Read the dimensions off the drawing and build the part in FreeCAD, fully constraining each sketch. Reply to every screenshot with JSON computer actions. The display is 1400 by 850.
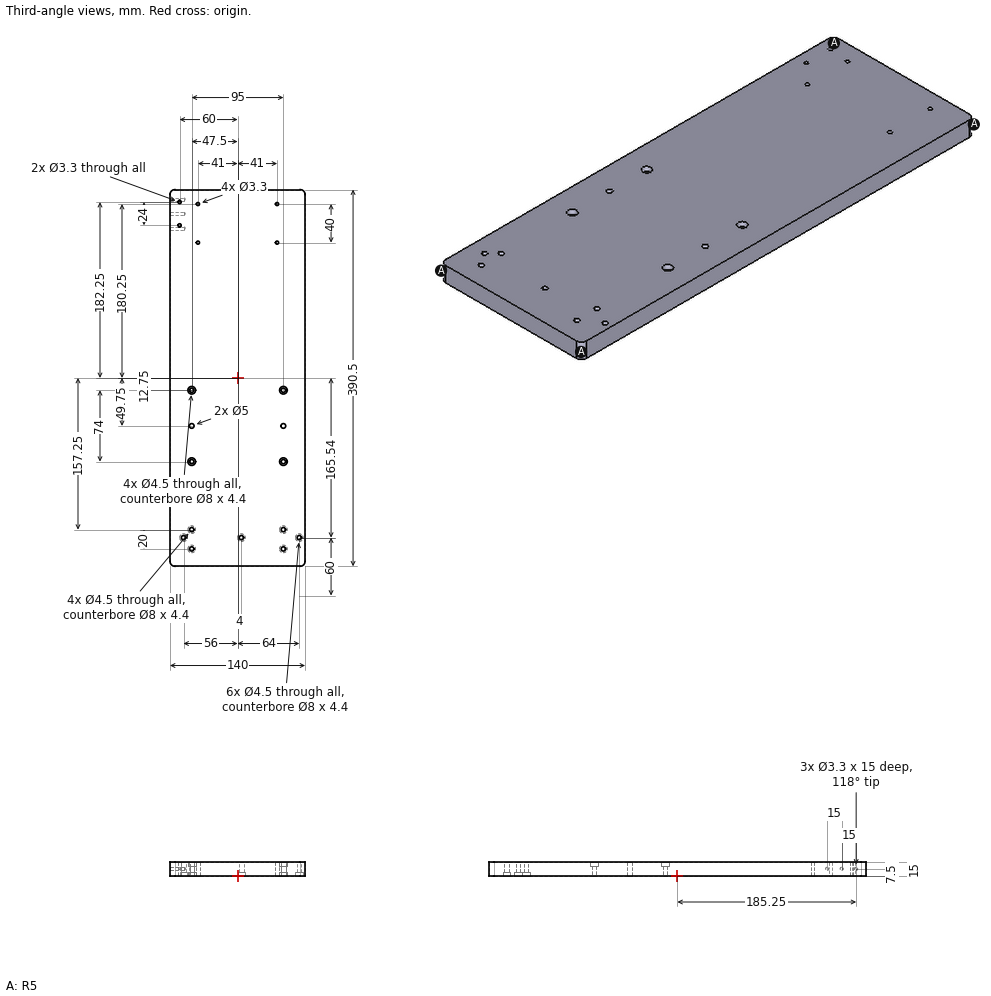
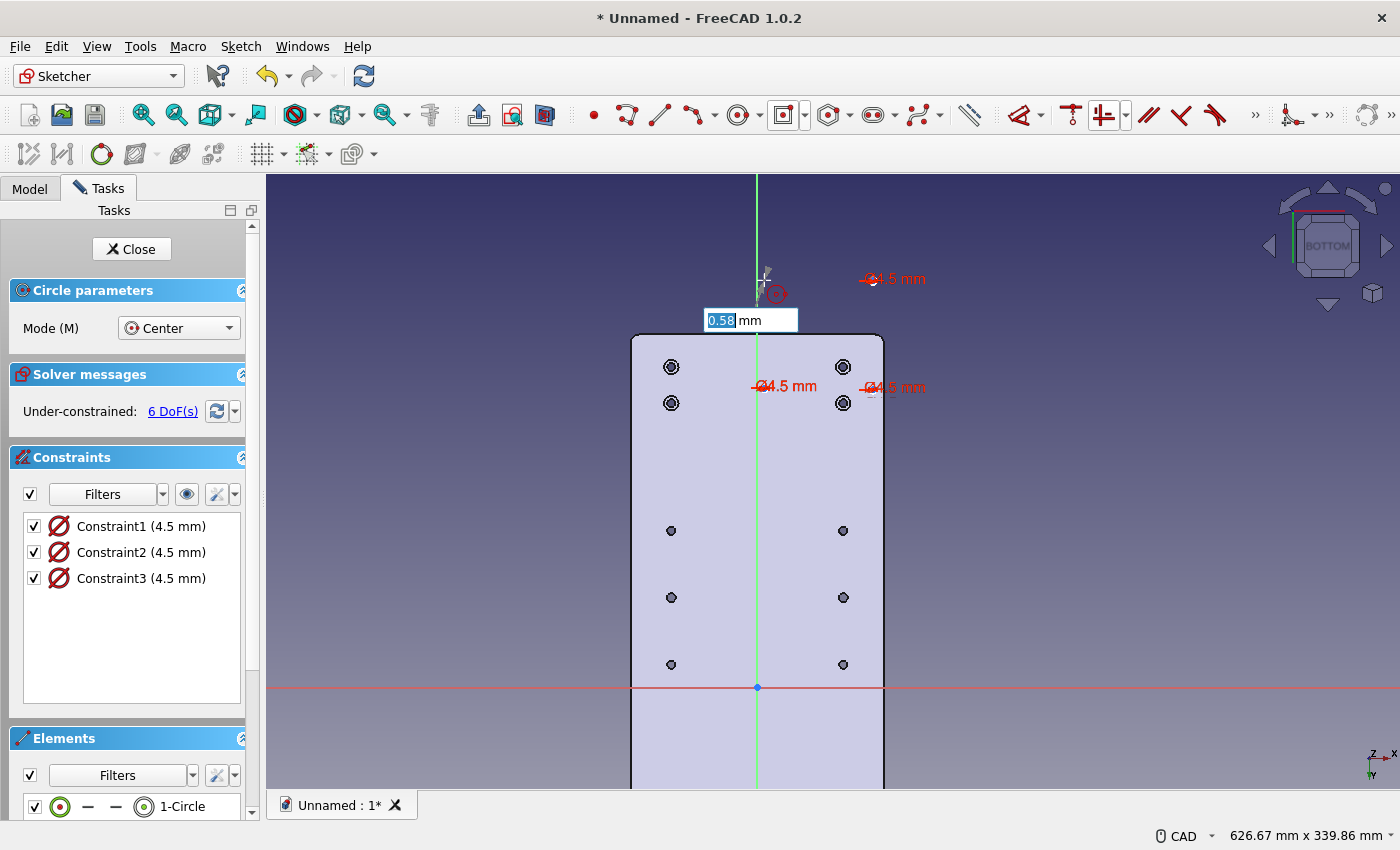
{"action": "scroll", "coordinate": [767, 277], "scroll_direction": "up", "scroll_amount": 3}
{"action": "mouse_move", "coordinate": [767, 276]}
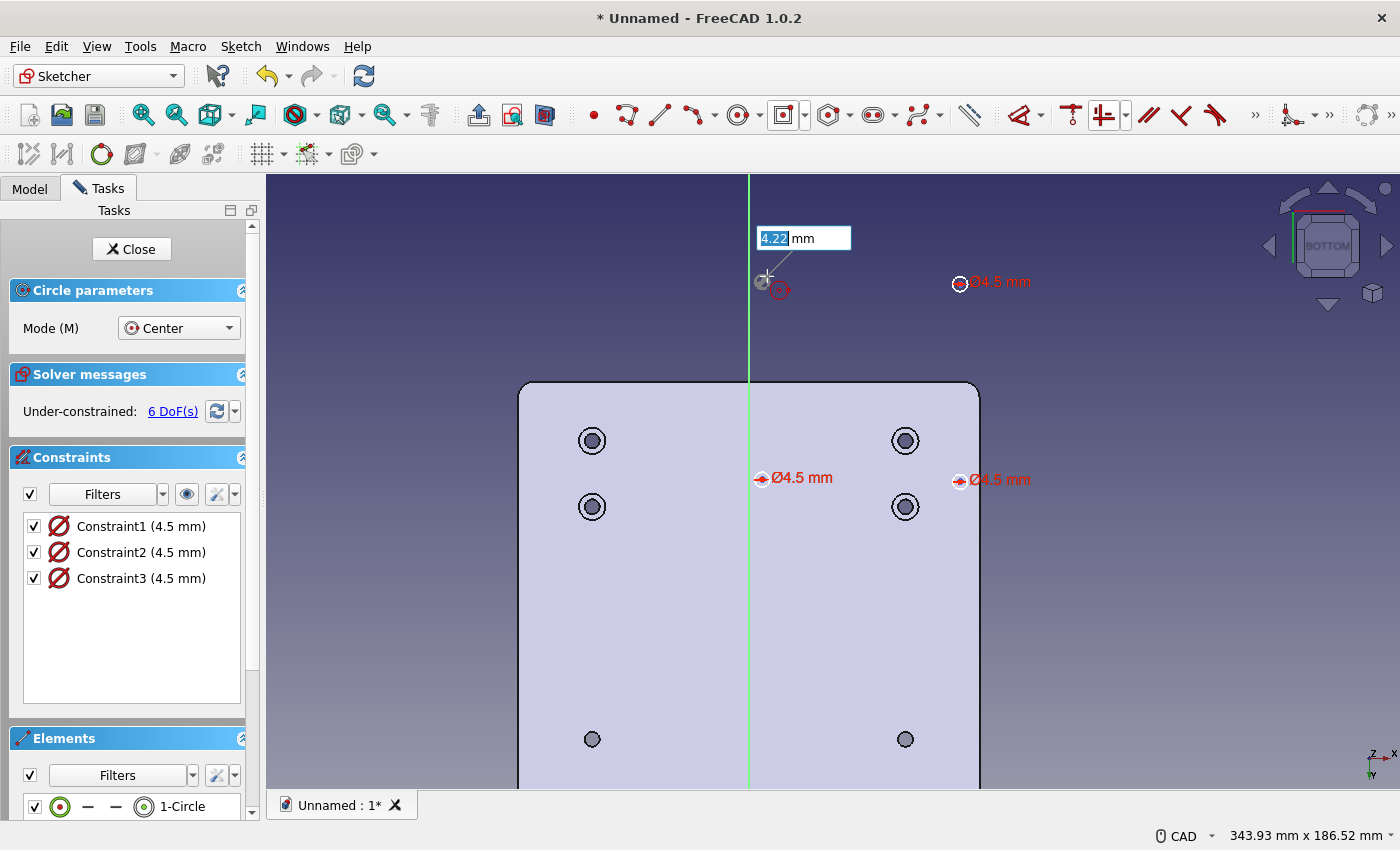
{"action": "type", "text": "4.5"}
{"action": "key", "text": "Return"}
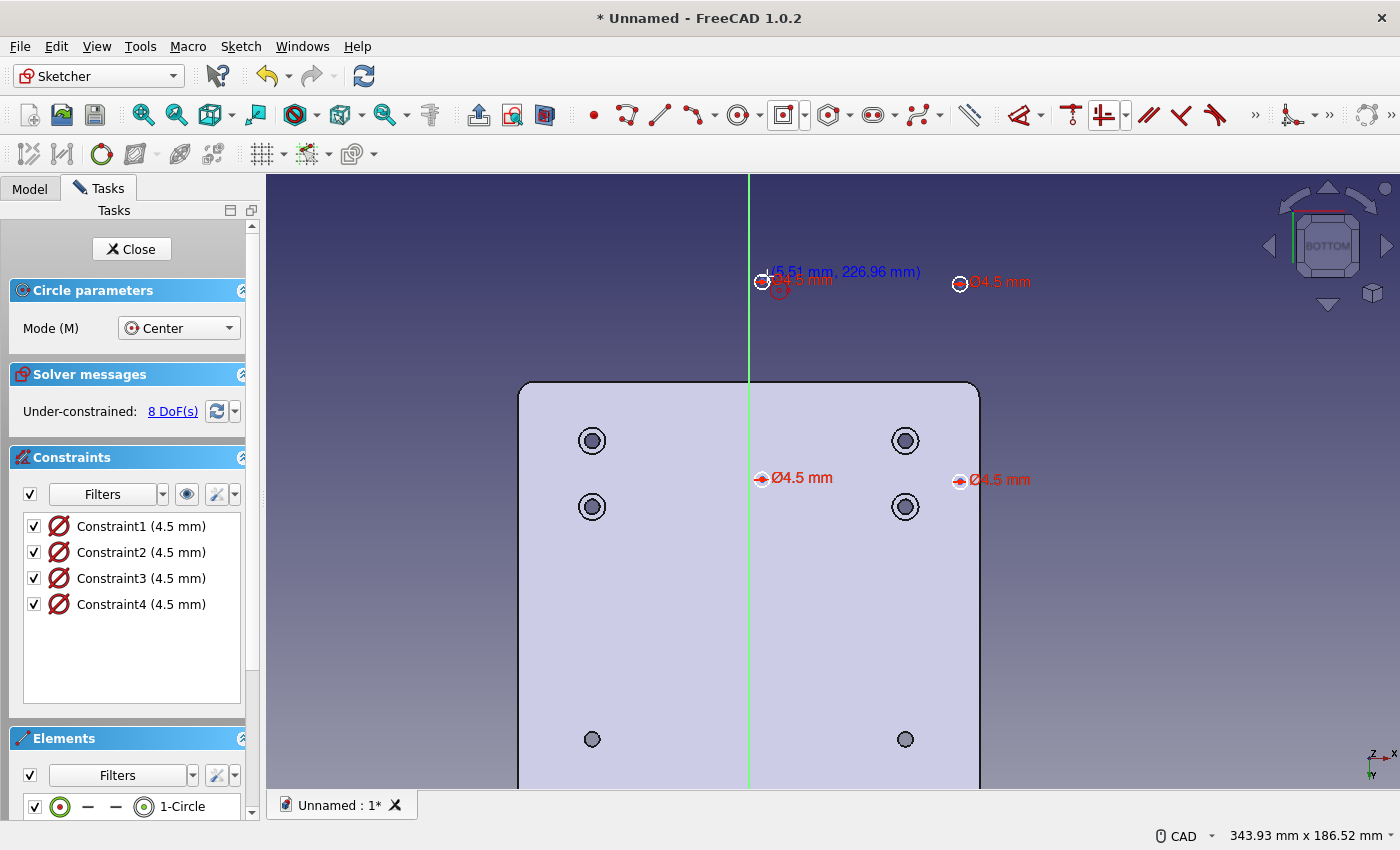
{"action": "scroll", "coordinate": [564, 480], "scroll_direction": "up", "scroll_amount": 6}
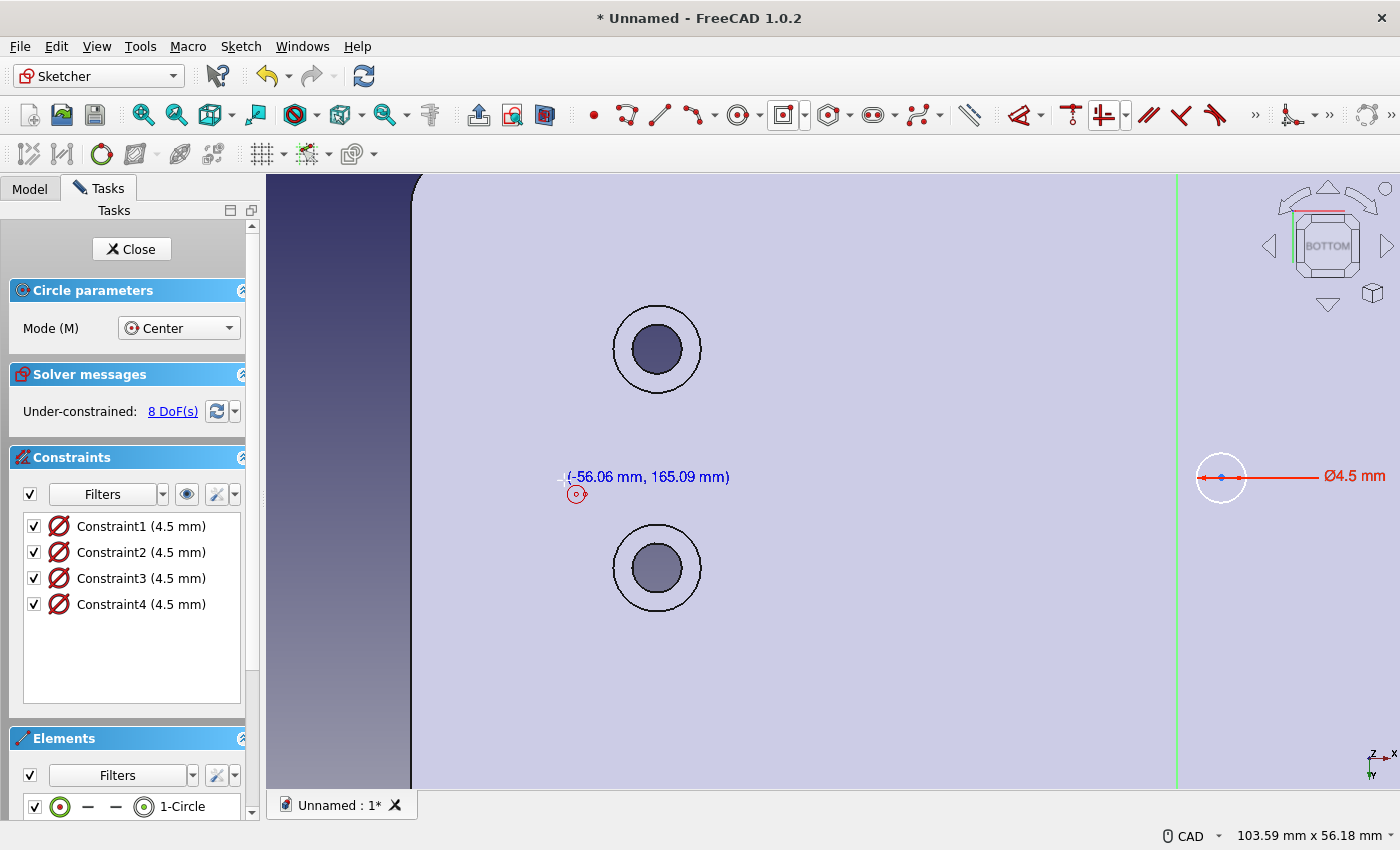
{"action": "scroll", "coordinate": [674, 370], "scroll_direction": "down", "scroll_amount": 9}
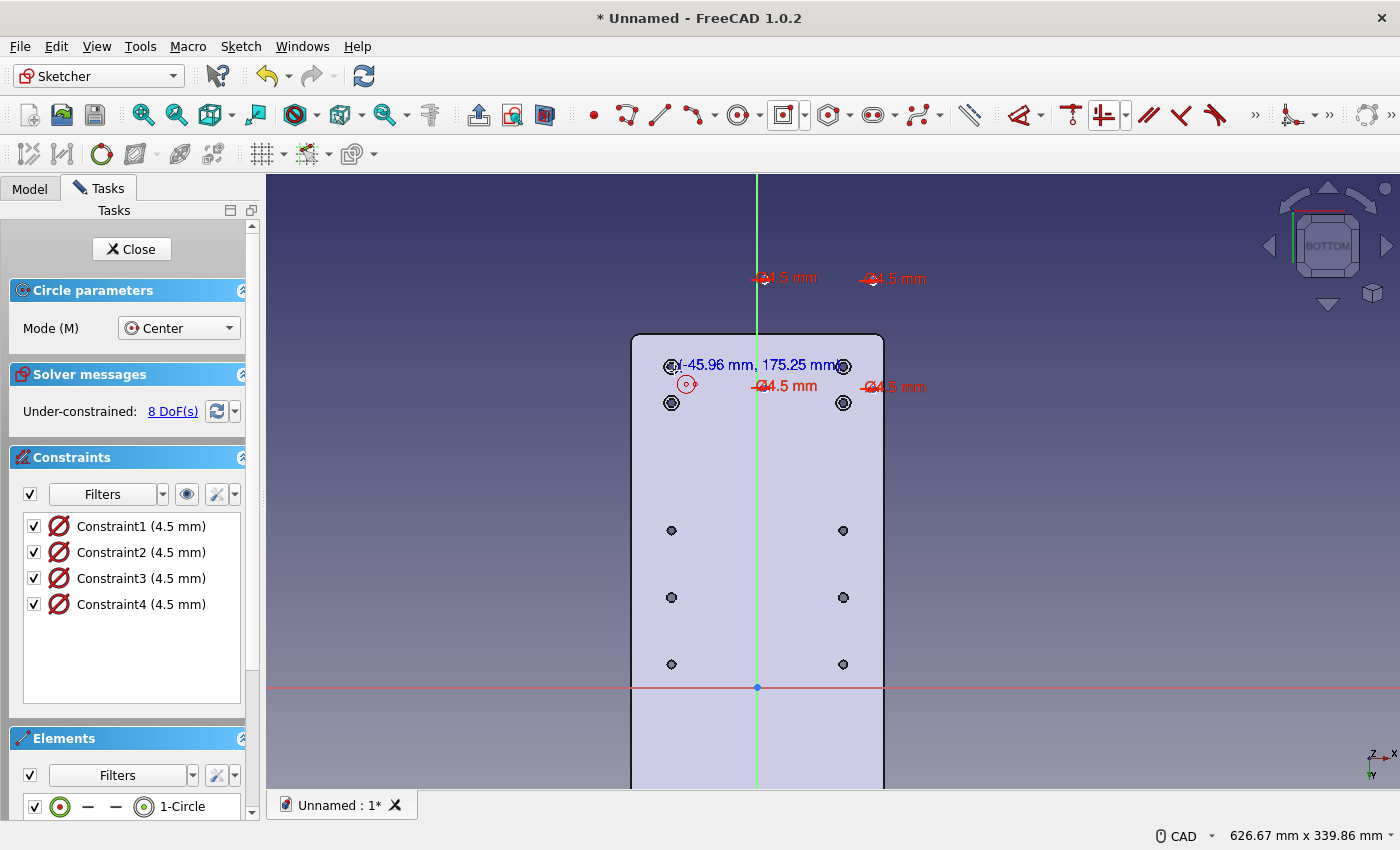
{"action": "left_click", "coordinate": [656, 388]}
{"action": "mouse_move", "coordinate": [659, 385]}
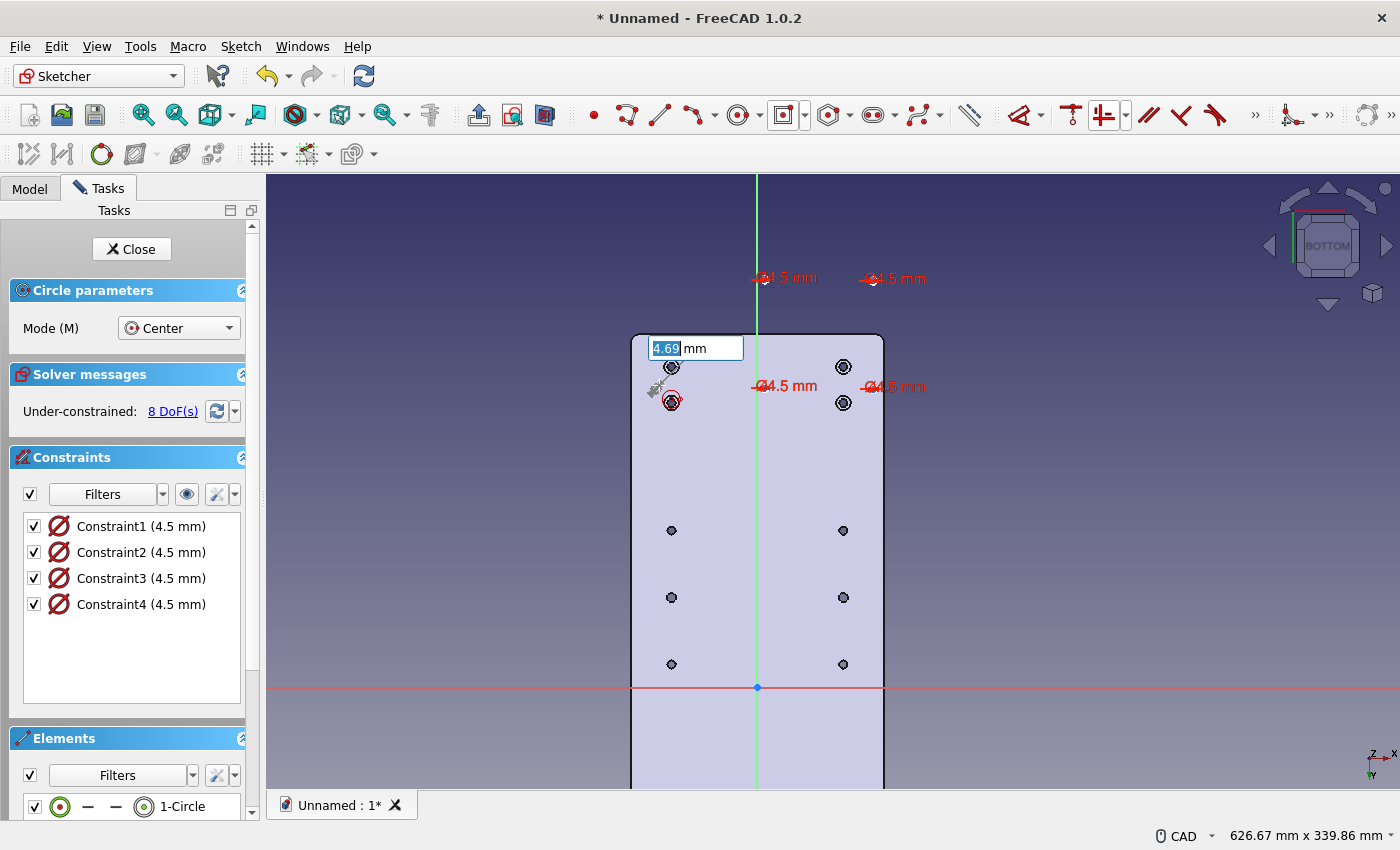
{"action": "type", "text": "4.5"}
{"action": "key", "text": "Return"}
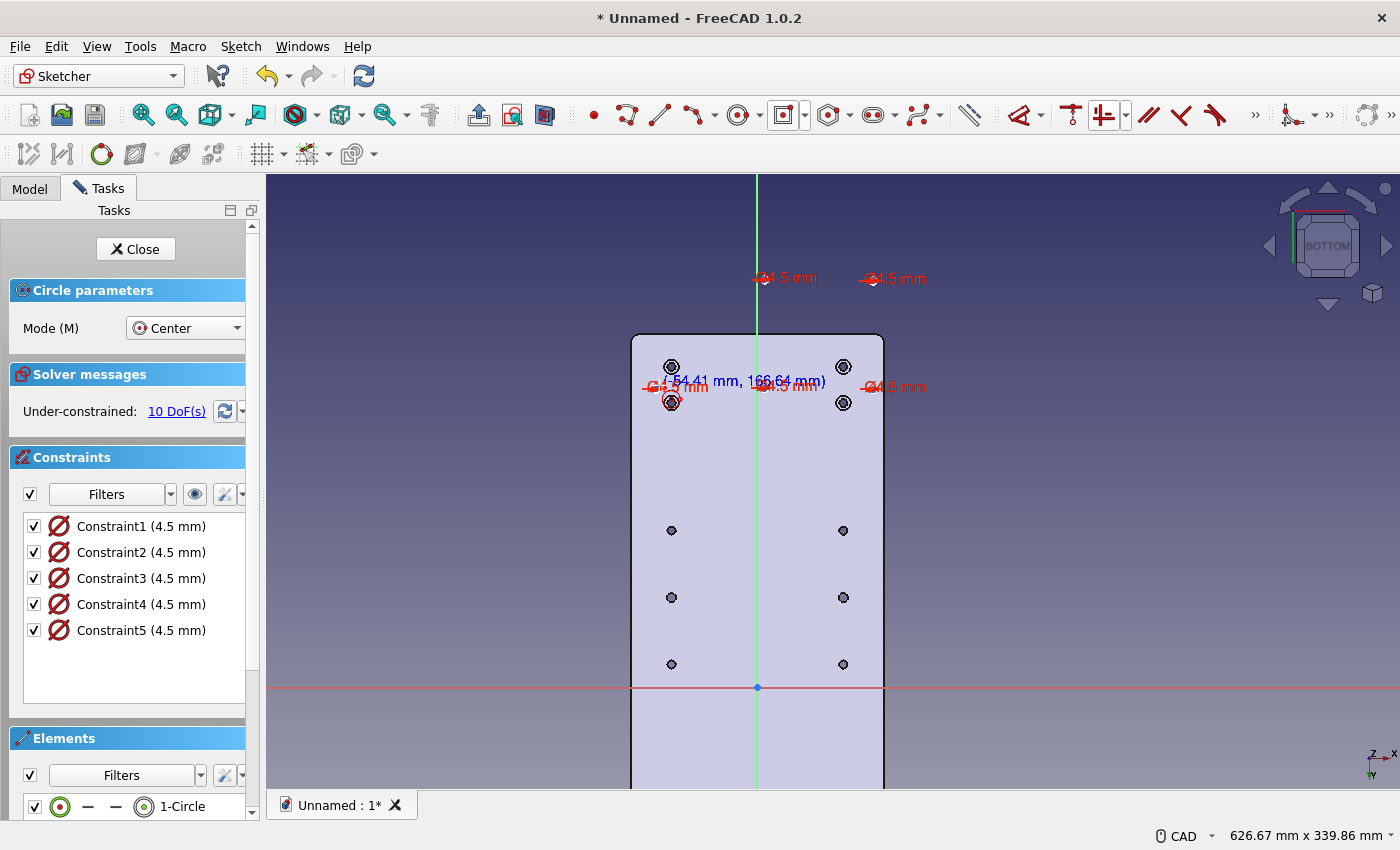
{"action": "scroll", "coordinate": [656, 279], "scroll_direction": "up", "scroll_amount": 9}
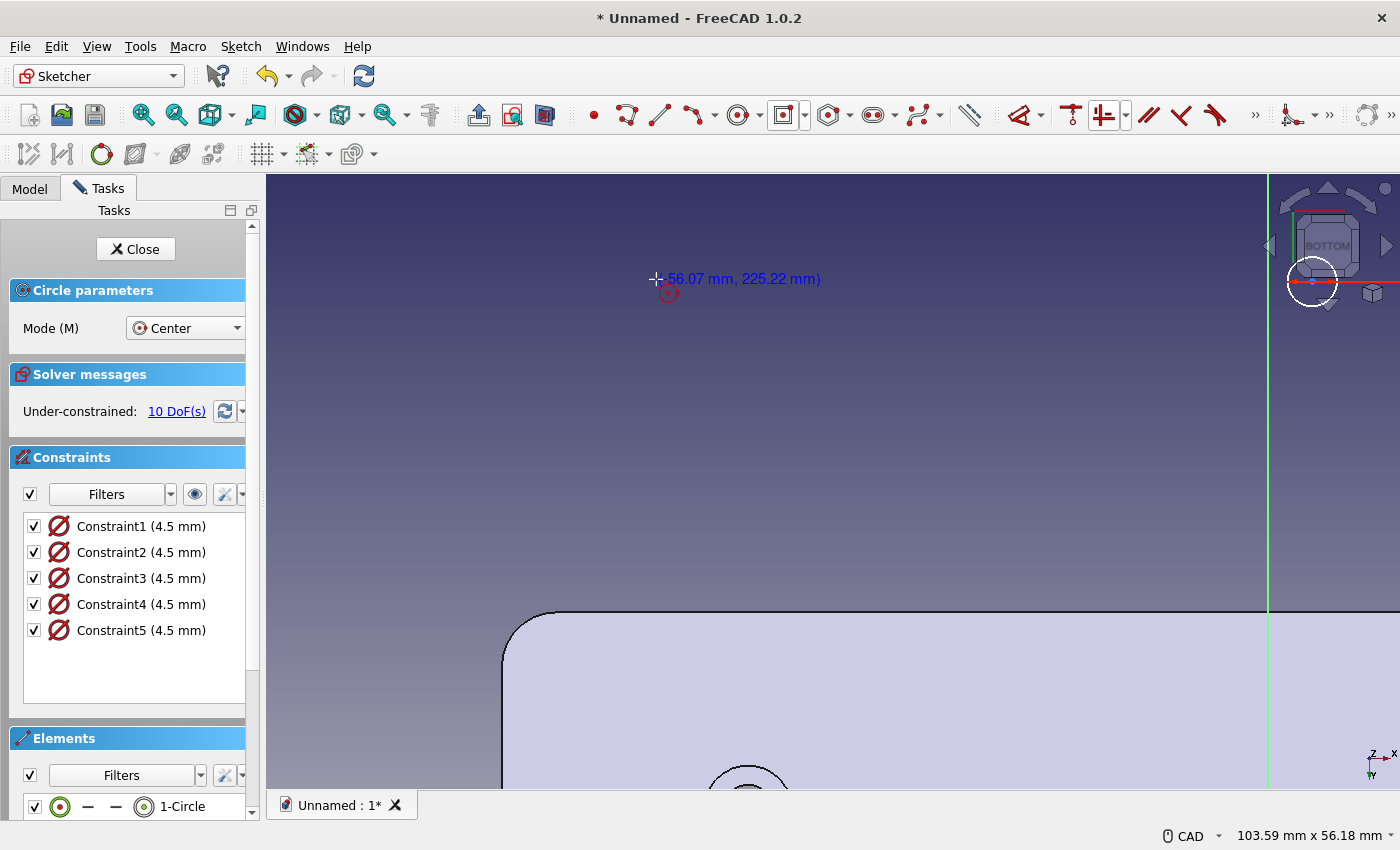
{"action": "scroll", "coordinate": [656, 279], "scroll_direction": "down", "scroll_amount": 9}